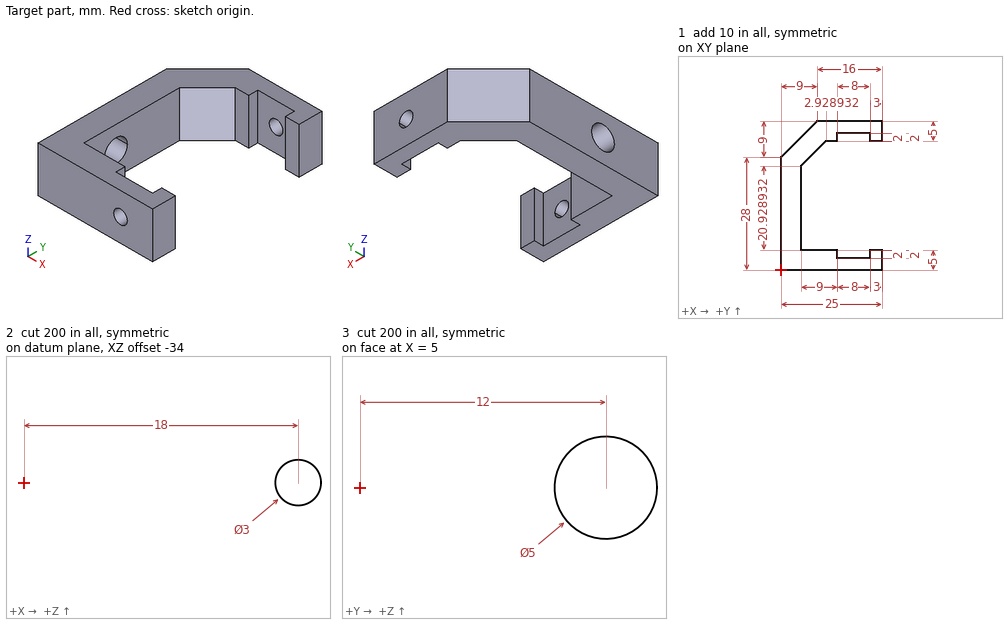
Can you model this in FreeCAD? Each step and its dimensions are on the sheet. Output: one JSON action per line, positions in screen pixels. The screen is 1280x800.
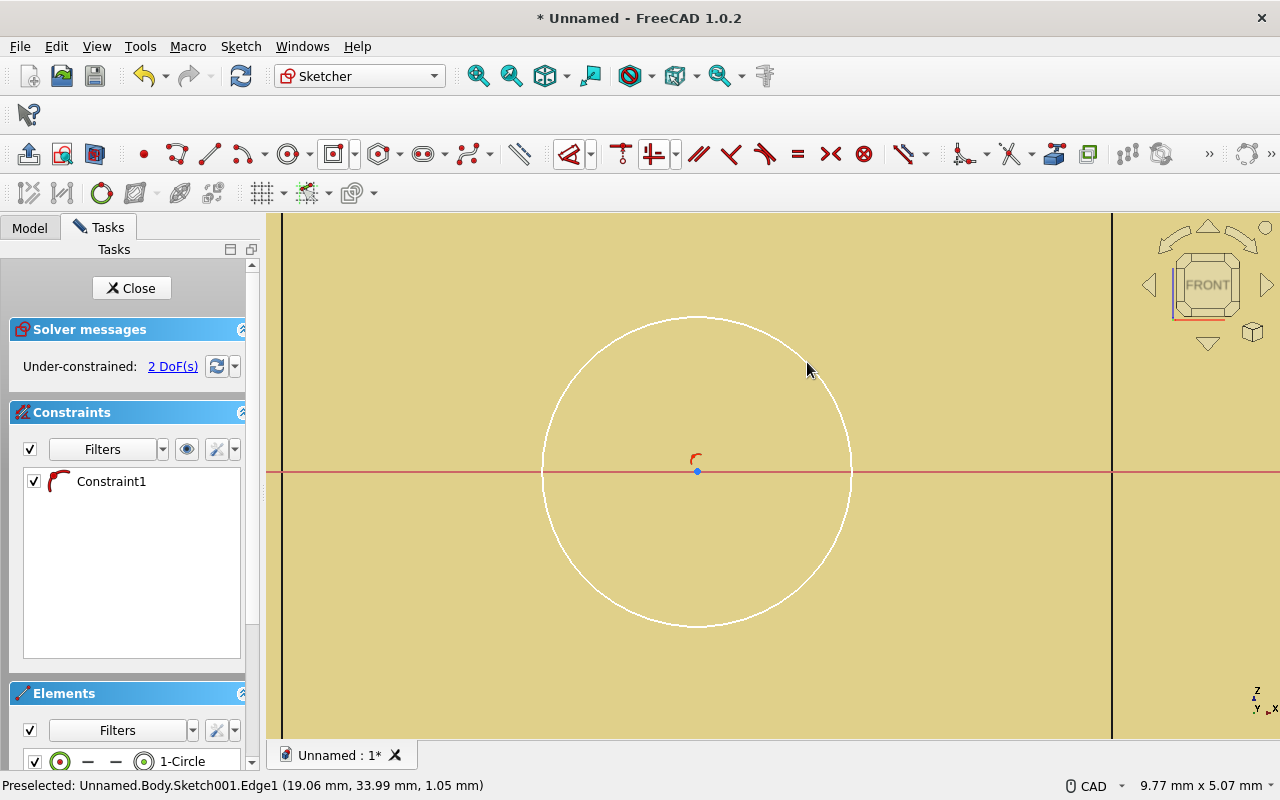
{"action": "left_click", "coordinate": [568, 154]}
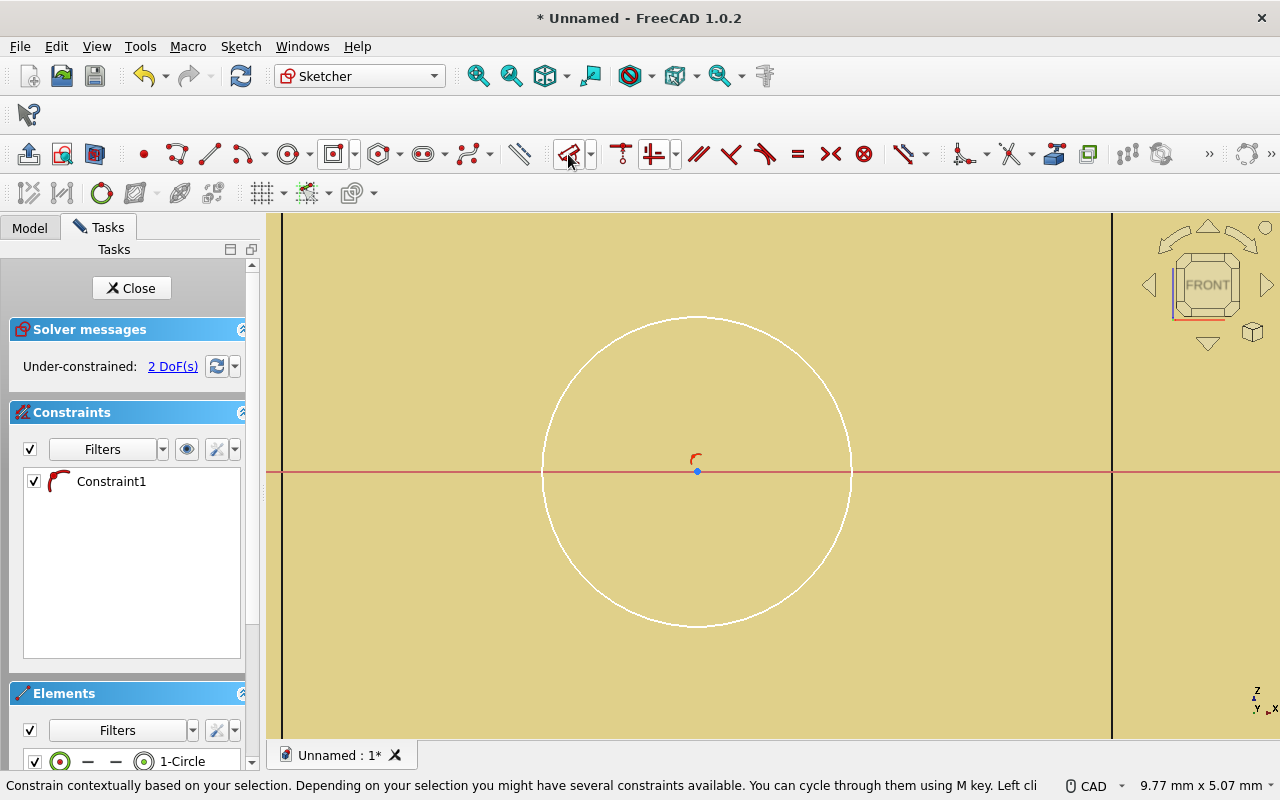
{"action": "left_click", "coordinate": [806, 362]}
{"action": "left_click", "coordinate": [829, 339]}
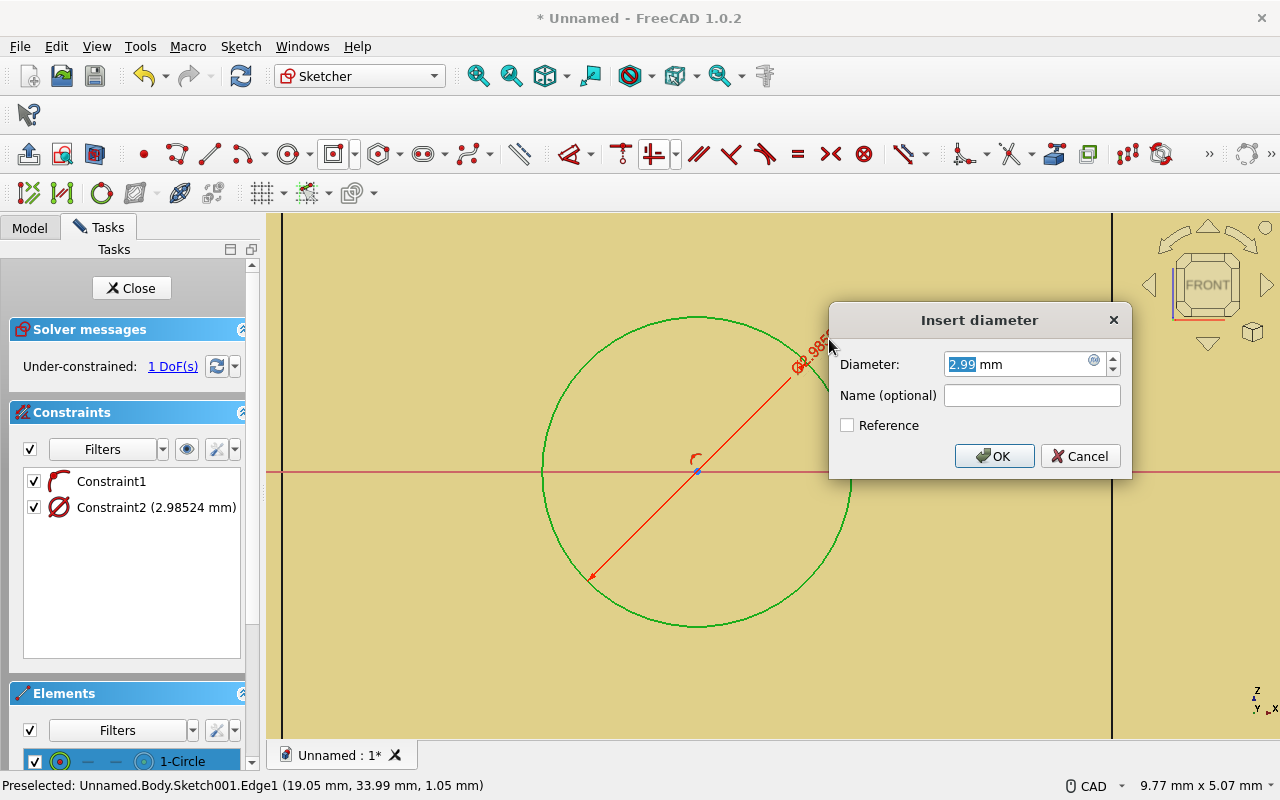
{"action": "type", "text": "3"}
{"action": "key", "text": "Return"}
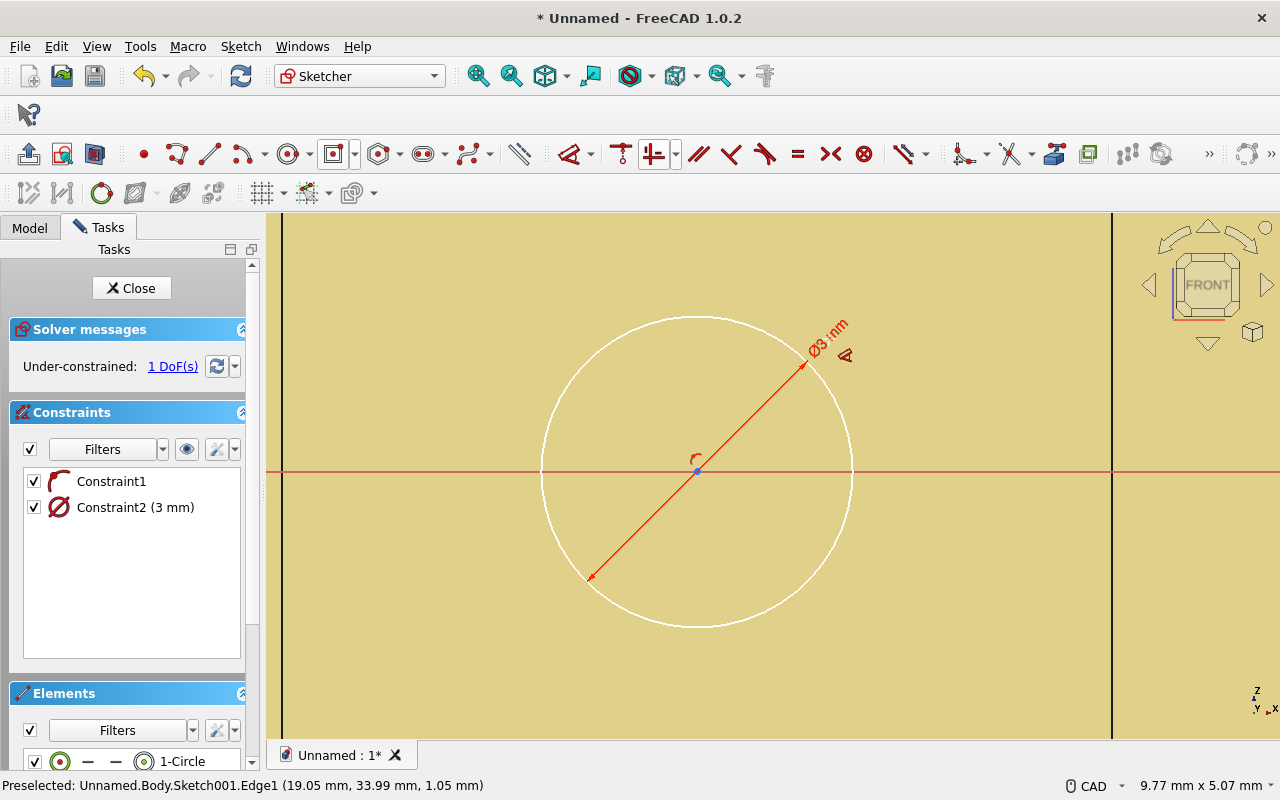
{"action": "left_click", "coordinate": [697, 472]}
{"action": "left_click", "coordinate": [495, 506]}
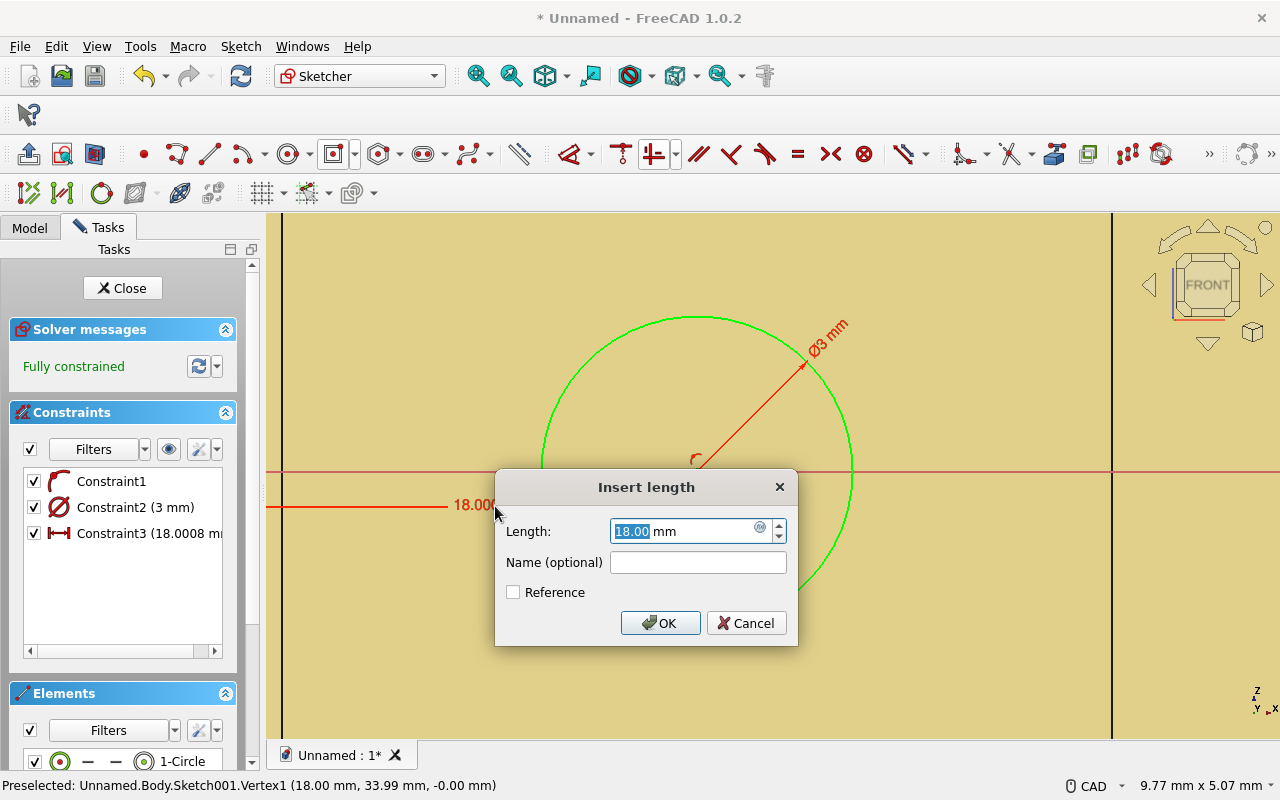
{"action": "type", "text": "18"}
{"action": "key", "text": "Return"}
{"action": "key", "text": "Escape"}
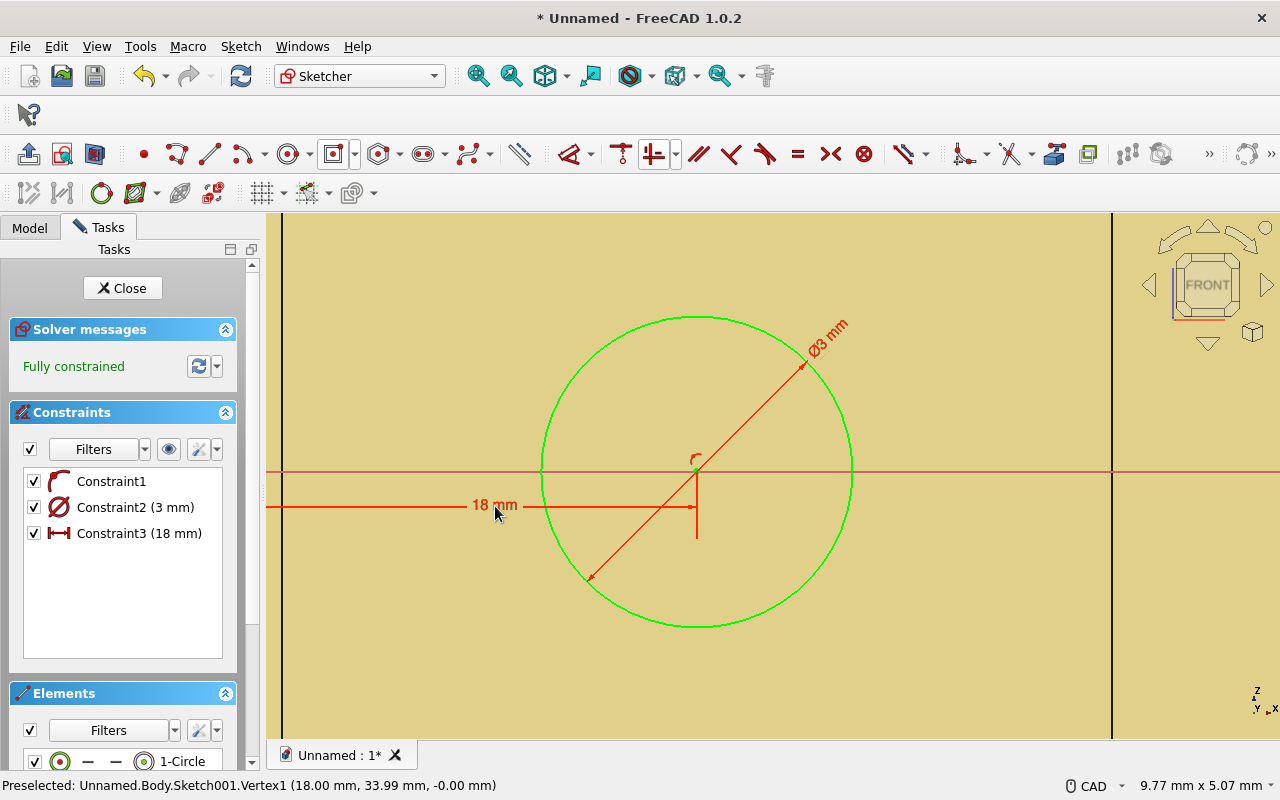
{"action": "left_click", "coordinate": [123, 288]}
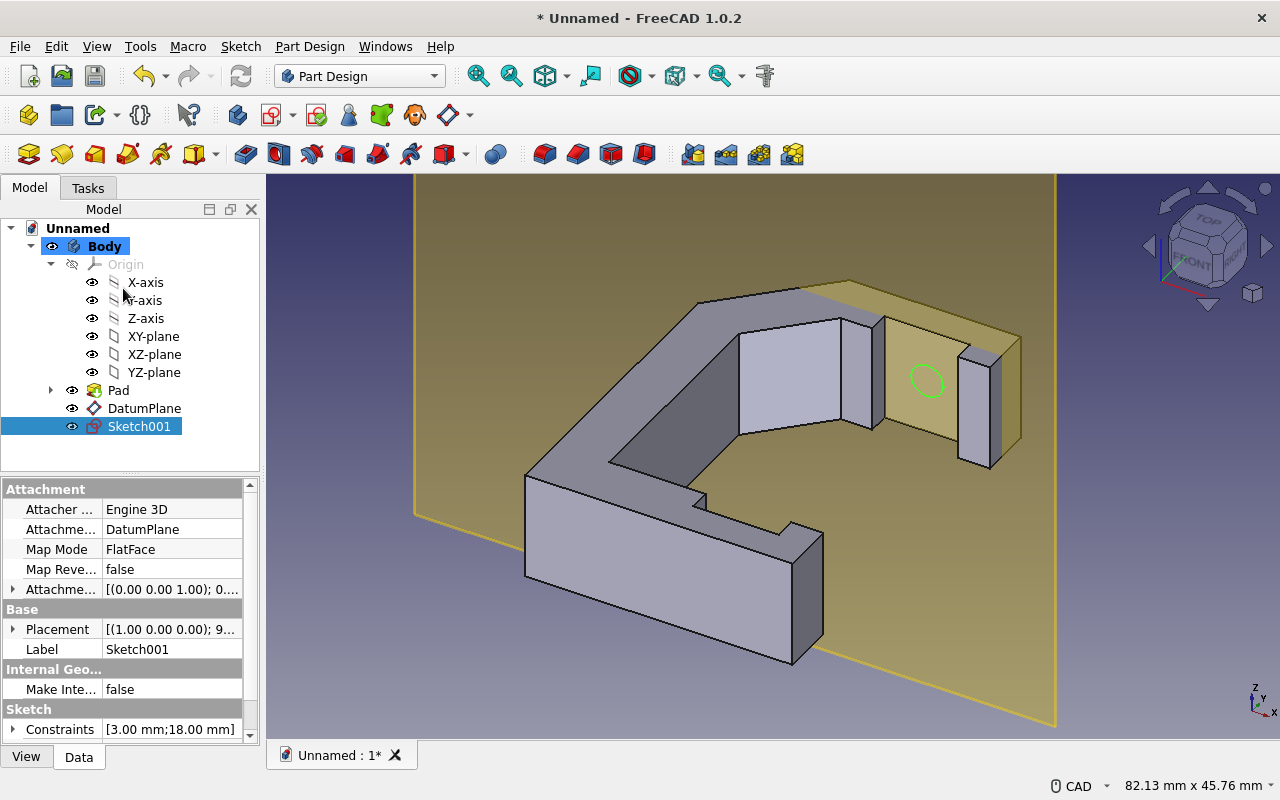
{"action": "left_click", "coordinate": [246, 154]}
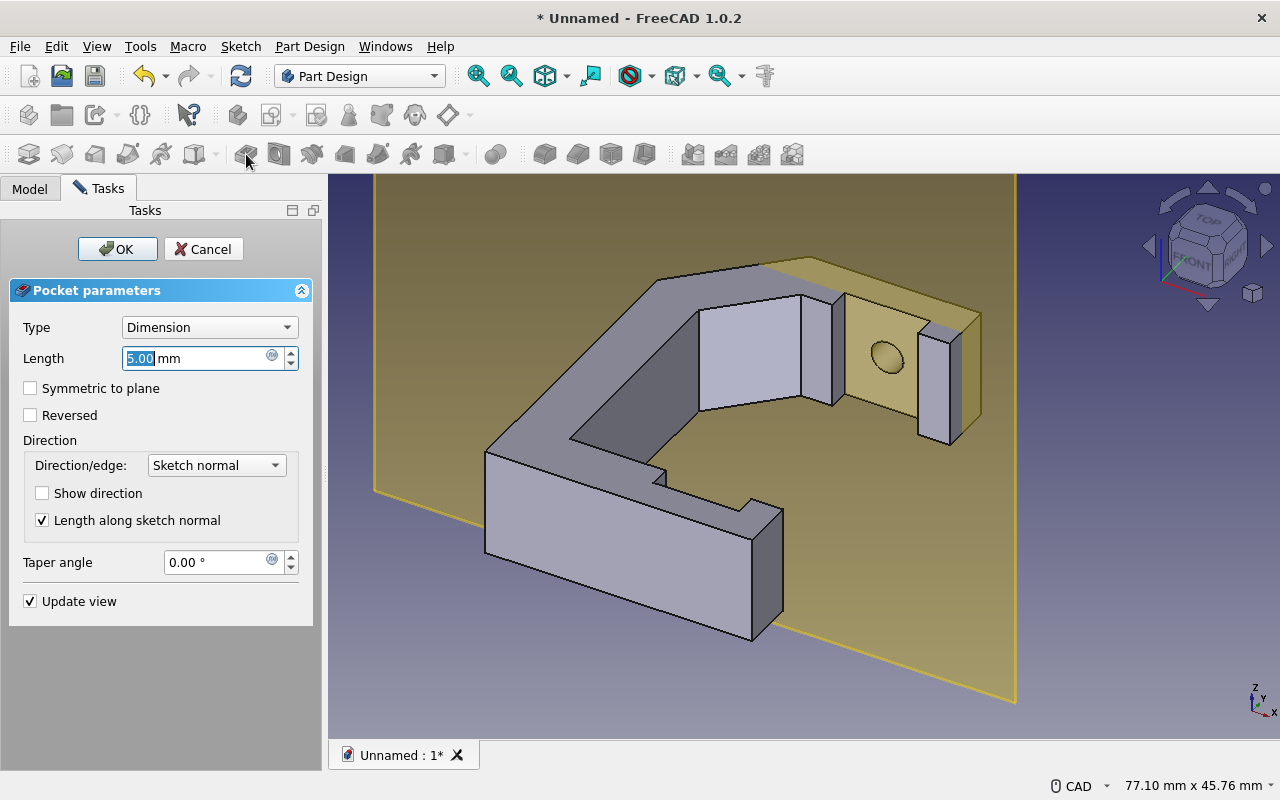
{"action": "type", "text": "200"}
{"action": "key", "text": "Tab"}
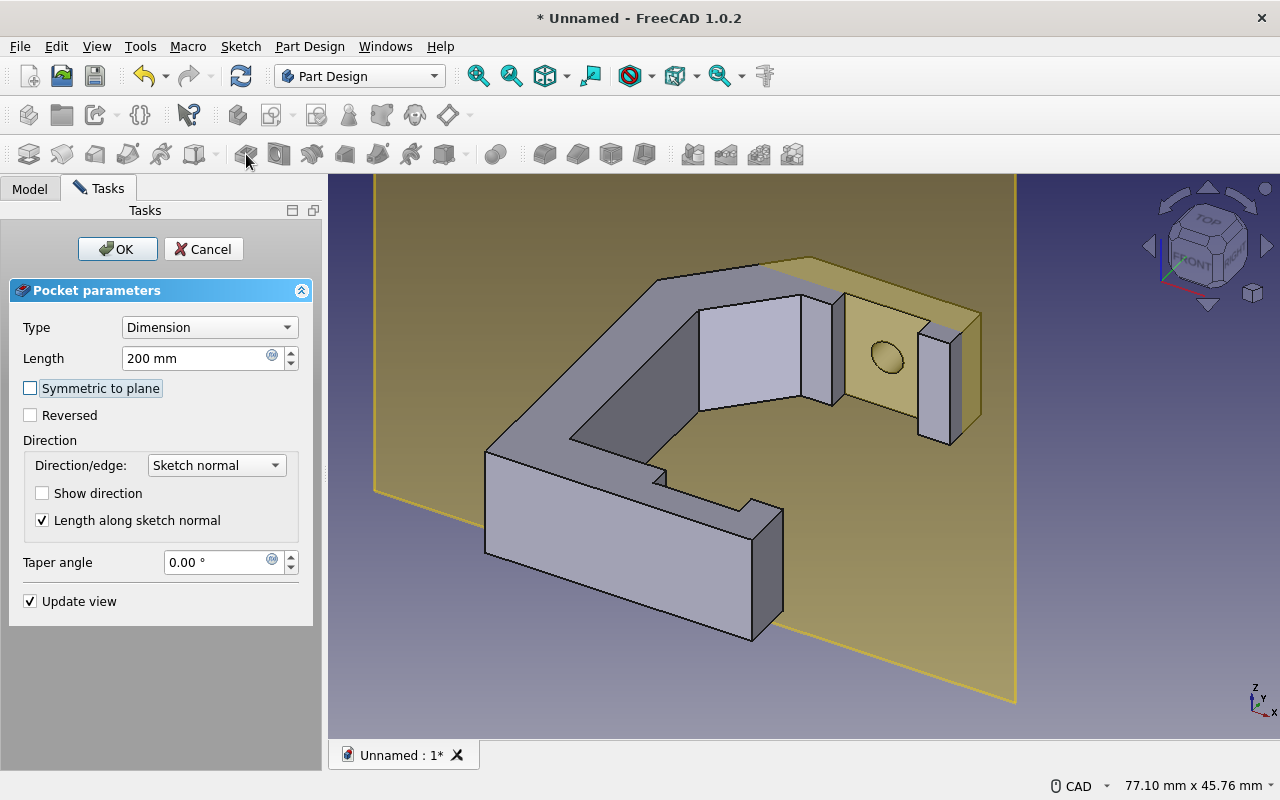
{"action": "left_click", "coordinate": [31, 388]}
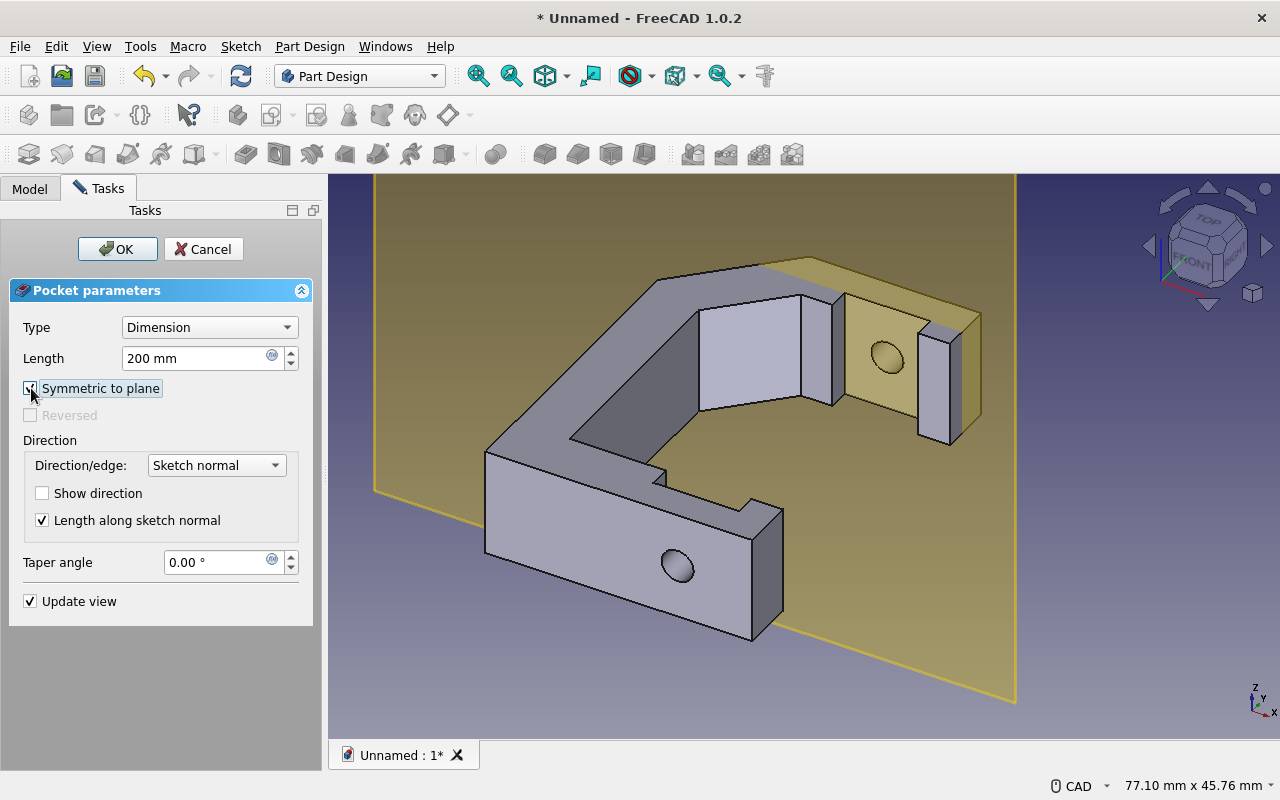
{"action": "left_click", "coordinate": [118, 249]}